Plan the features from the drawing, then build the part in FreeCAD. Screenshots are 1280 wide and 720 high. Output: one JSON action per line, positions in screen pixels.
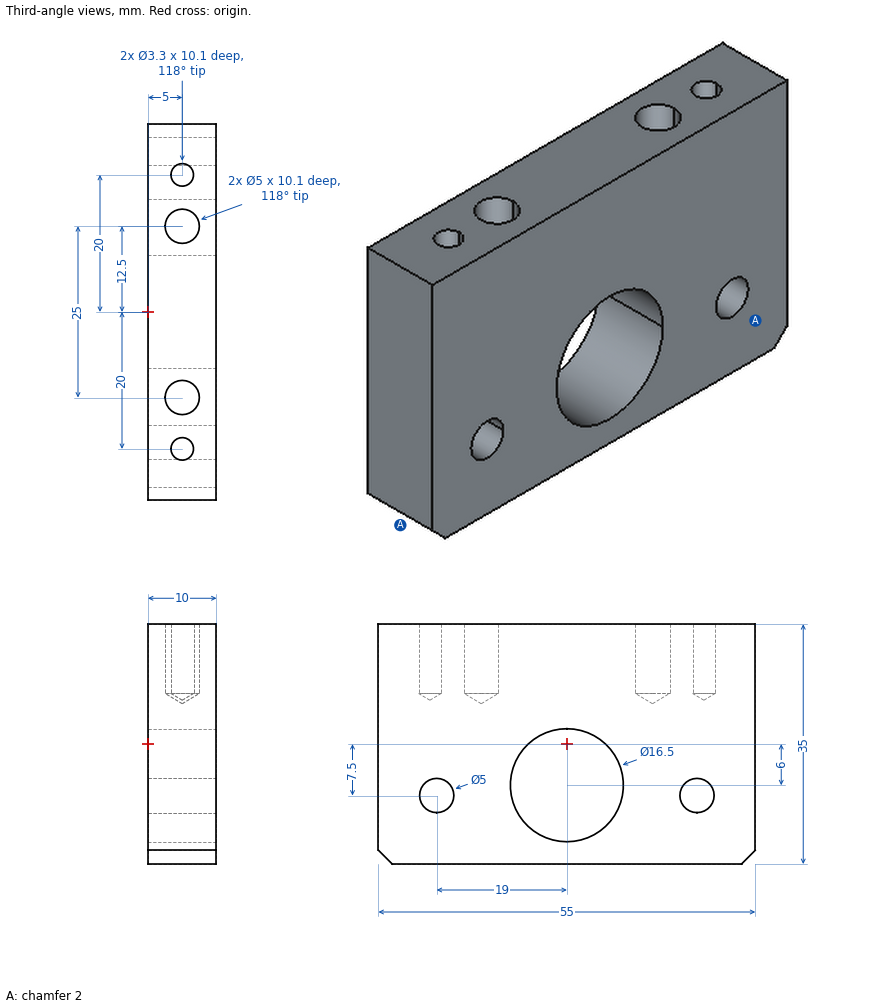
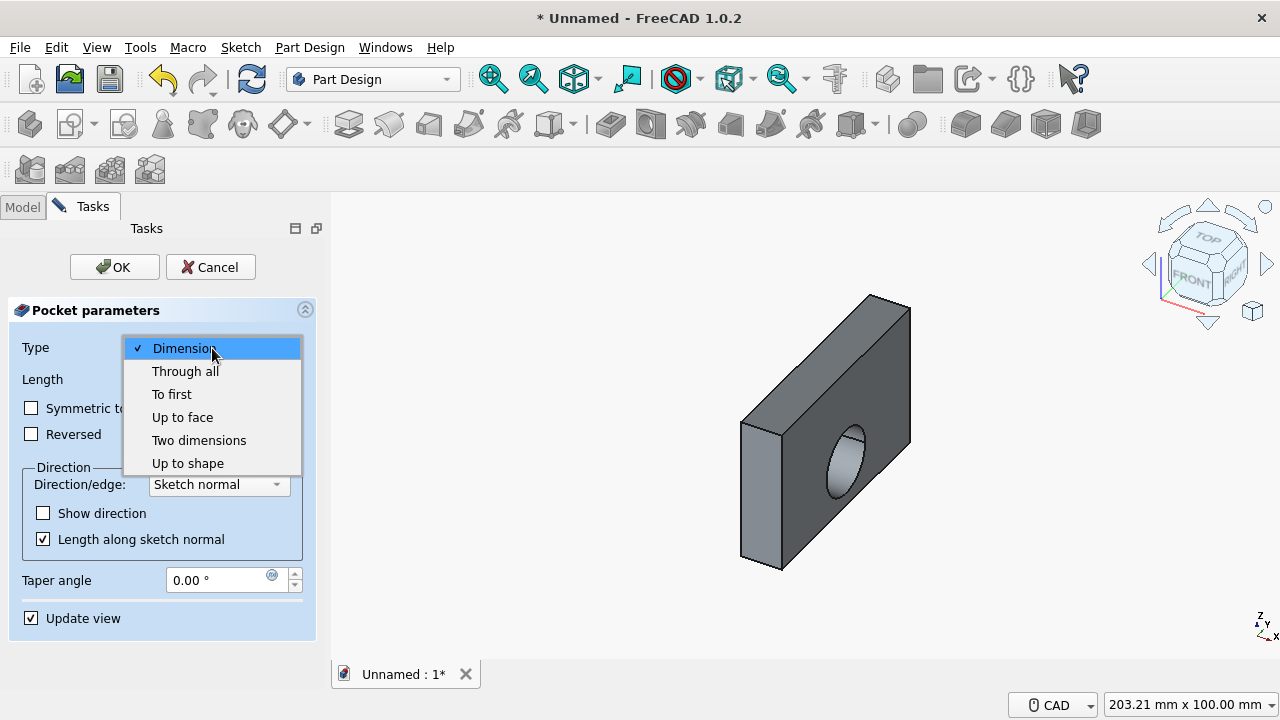
{"action": "left_click", "coordinate": [212, 372]}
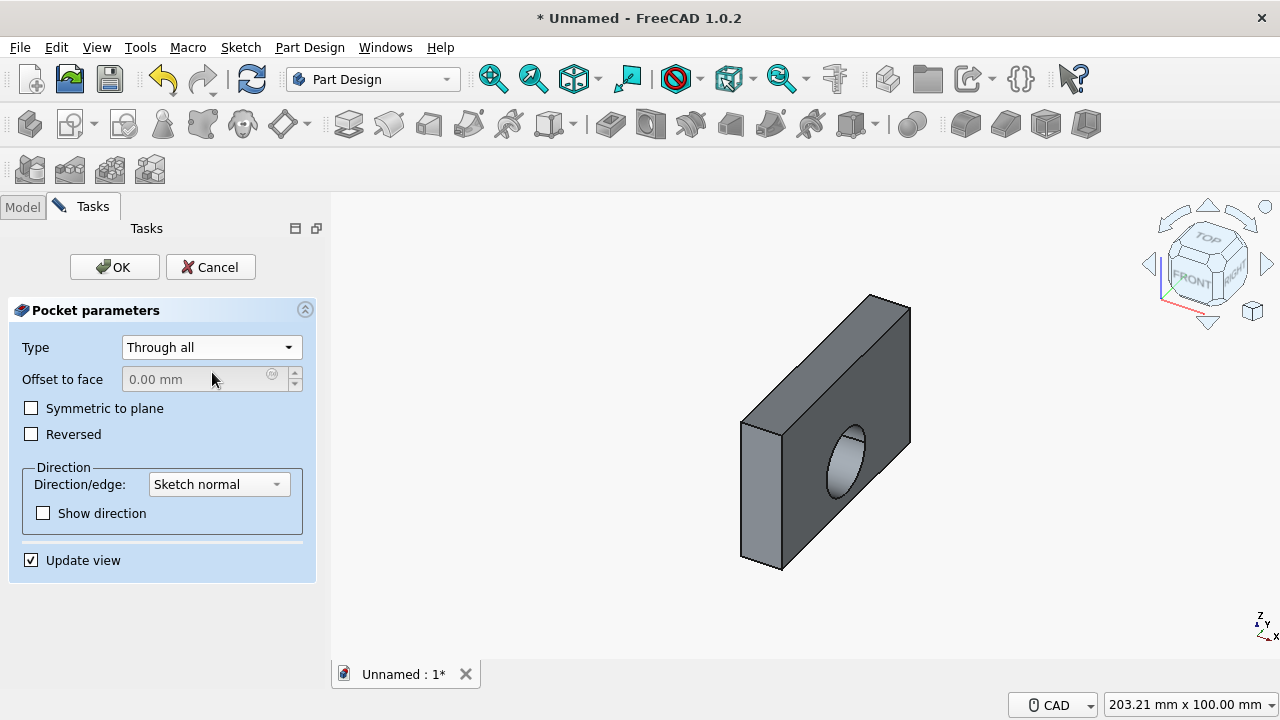
{"action": "left_click", "coordinate": [30, 434]}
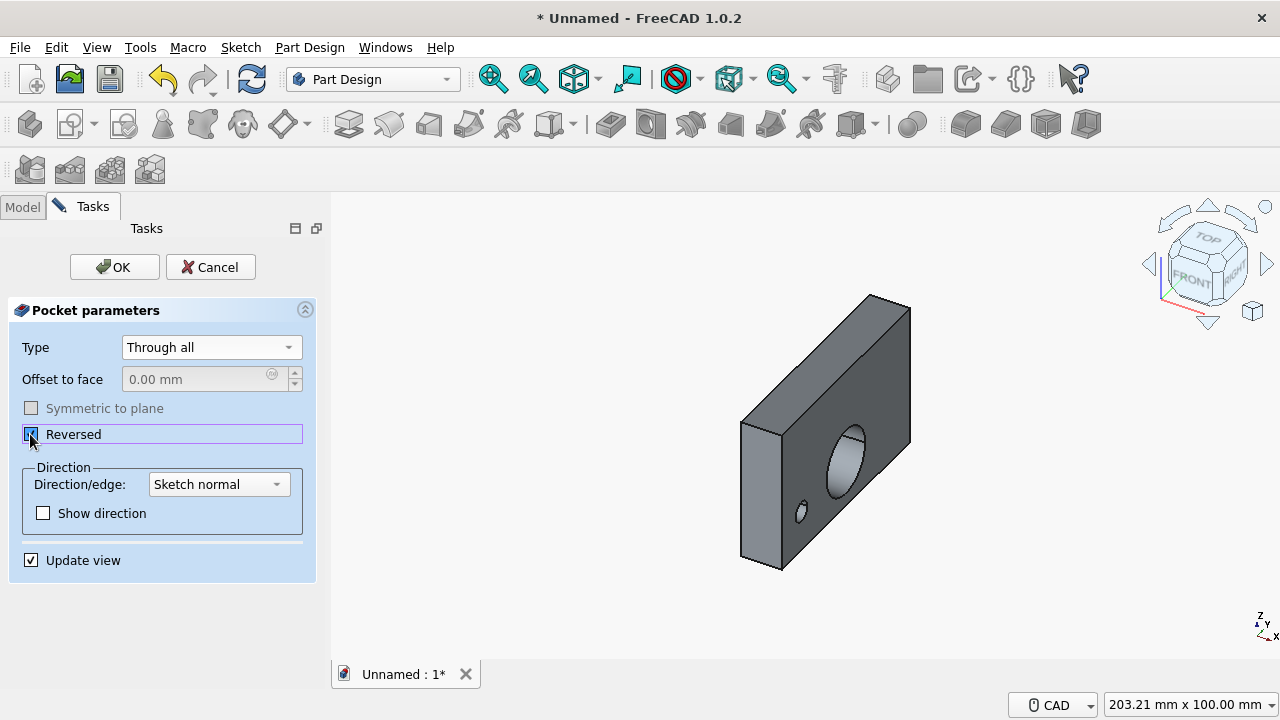
{"action": "left_click", "coordinate": [115, 267]}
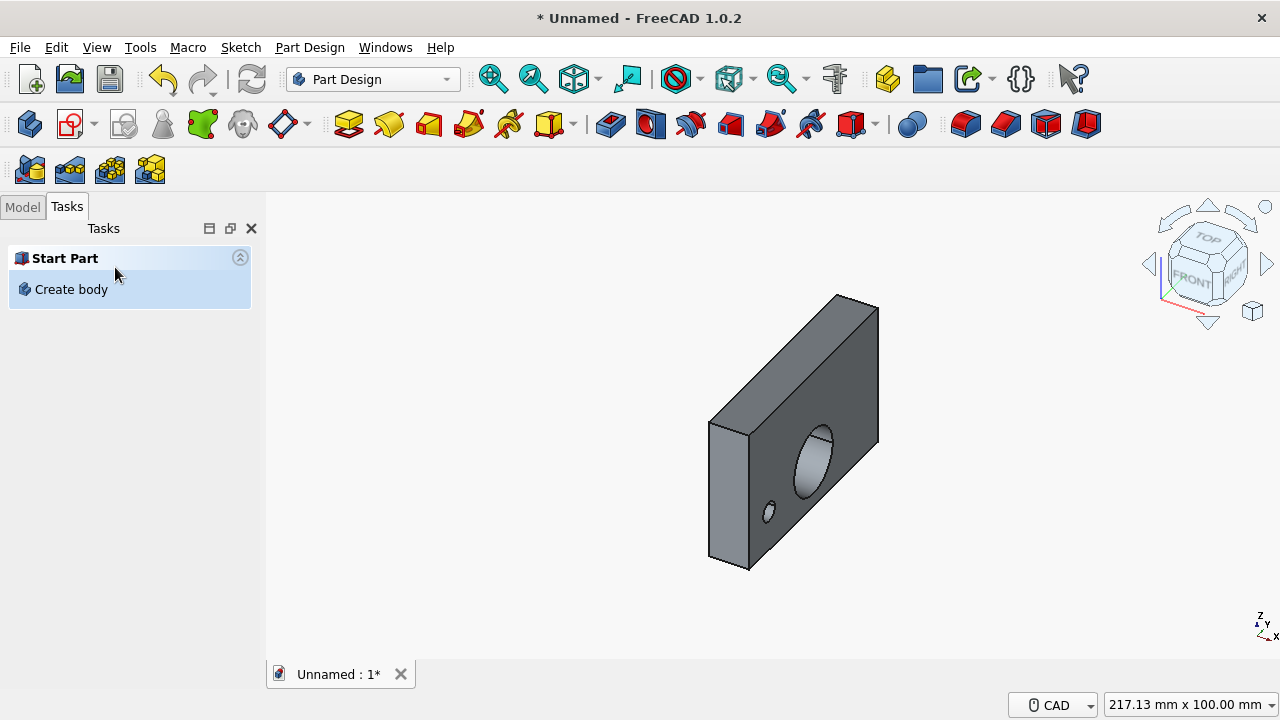
{"action": "left_click", "coordinate": [23, 206]}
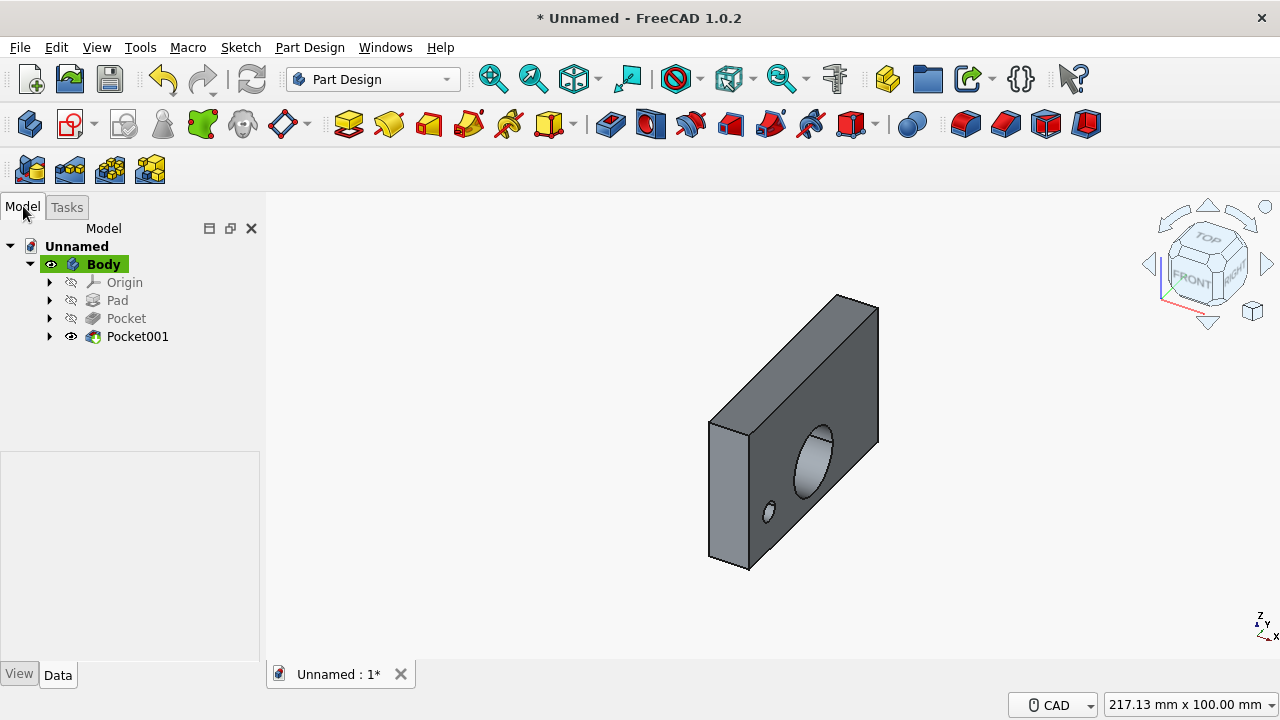
{"action": "left_click", "coordinate": [116, 336]}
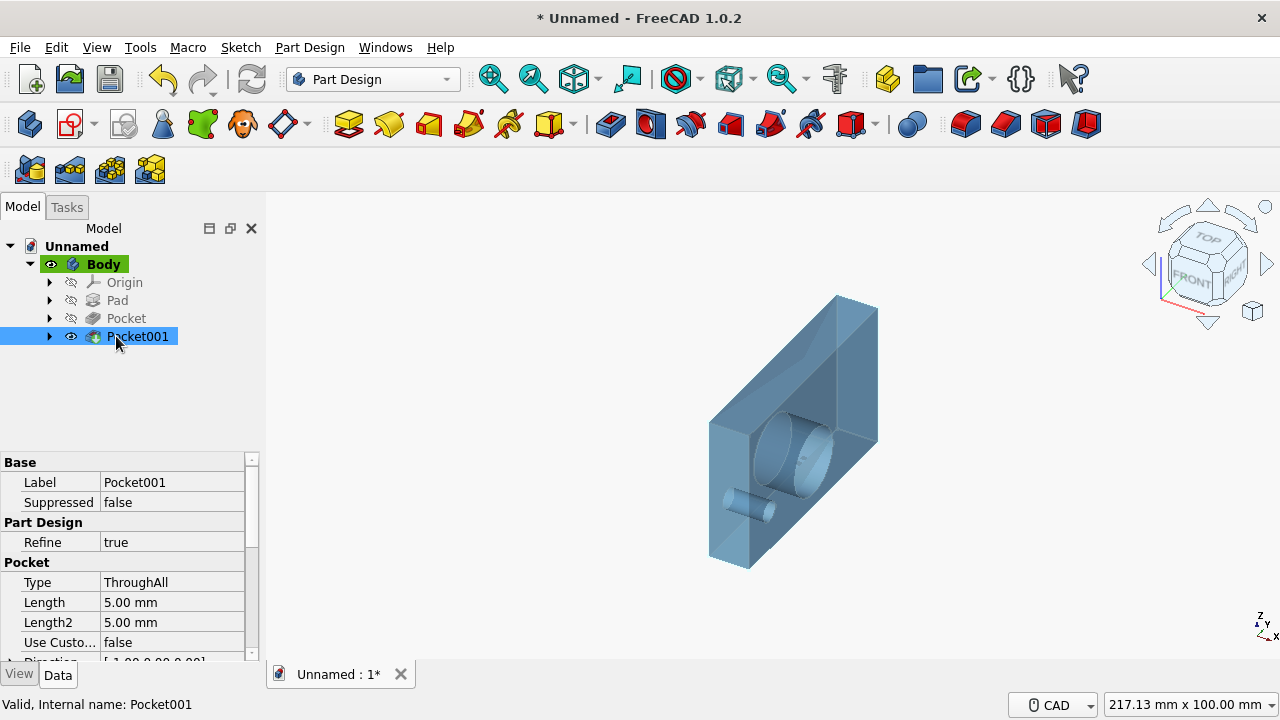
{"action": "left_click", "coordinate": [30, 170]}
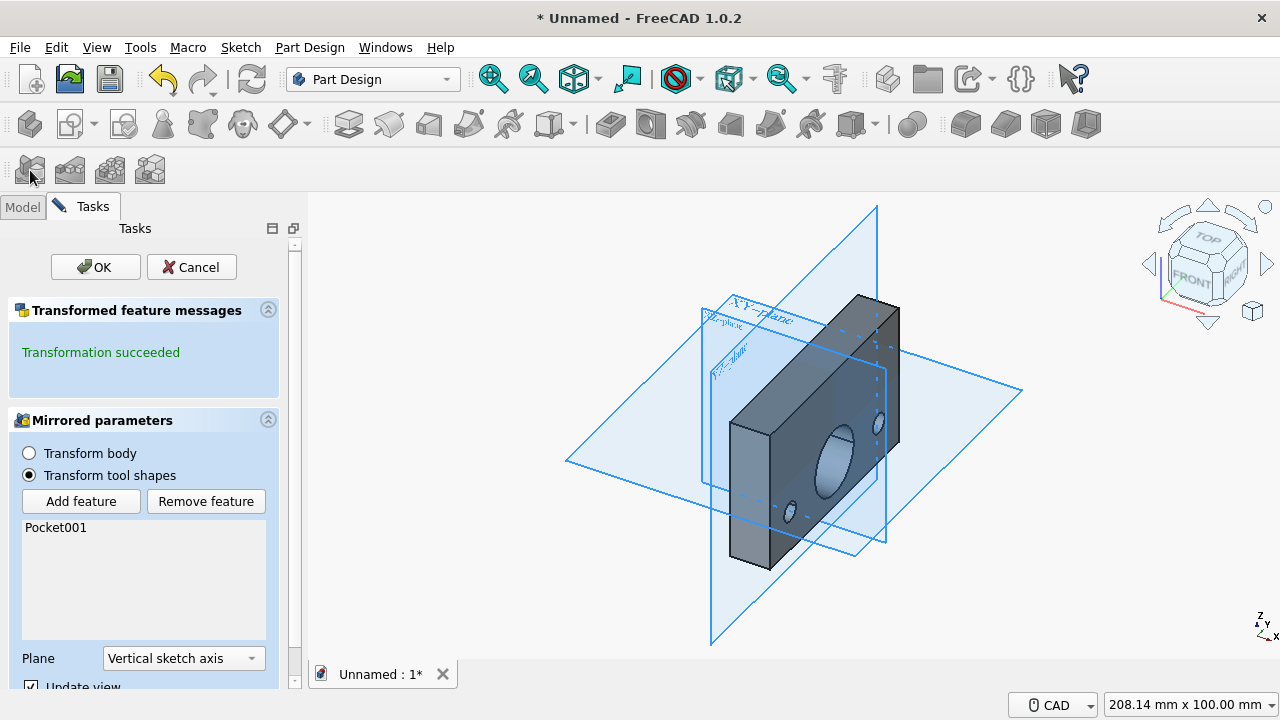
{"action": "left_click", "coordinate": [184, 658]}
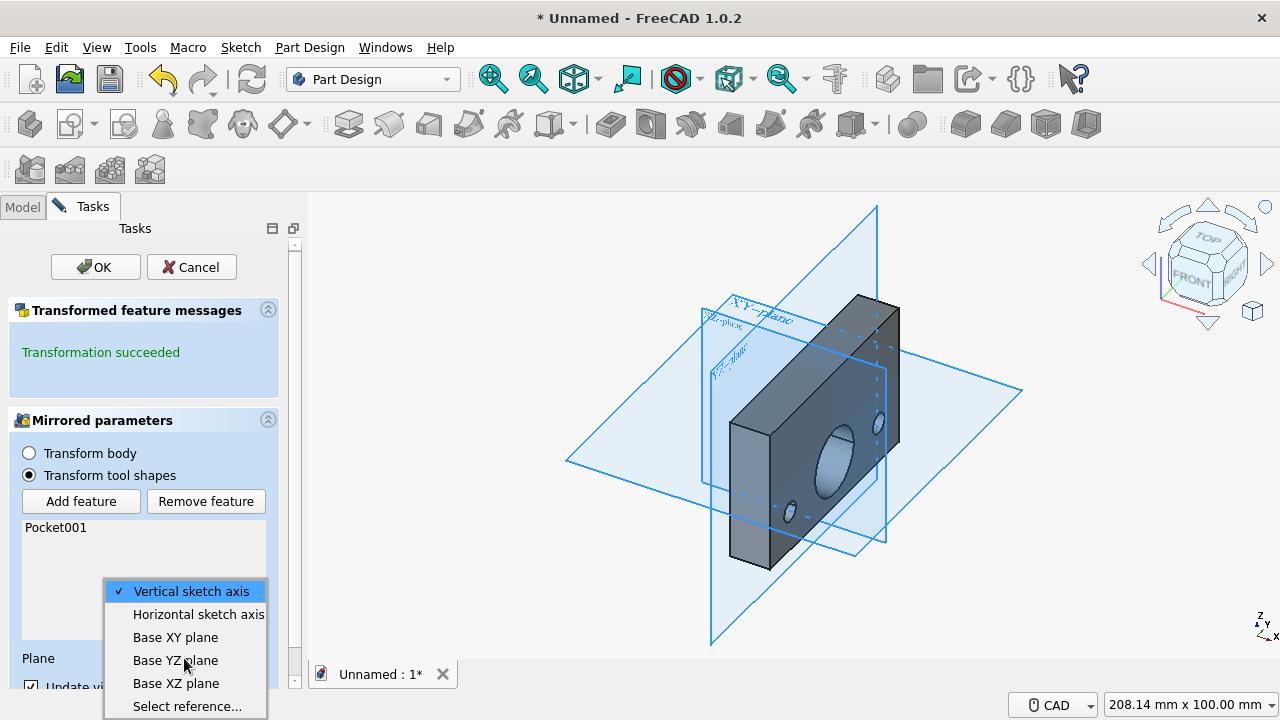
{"action": "left_click", "coordinate": [184, 684]}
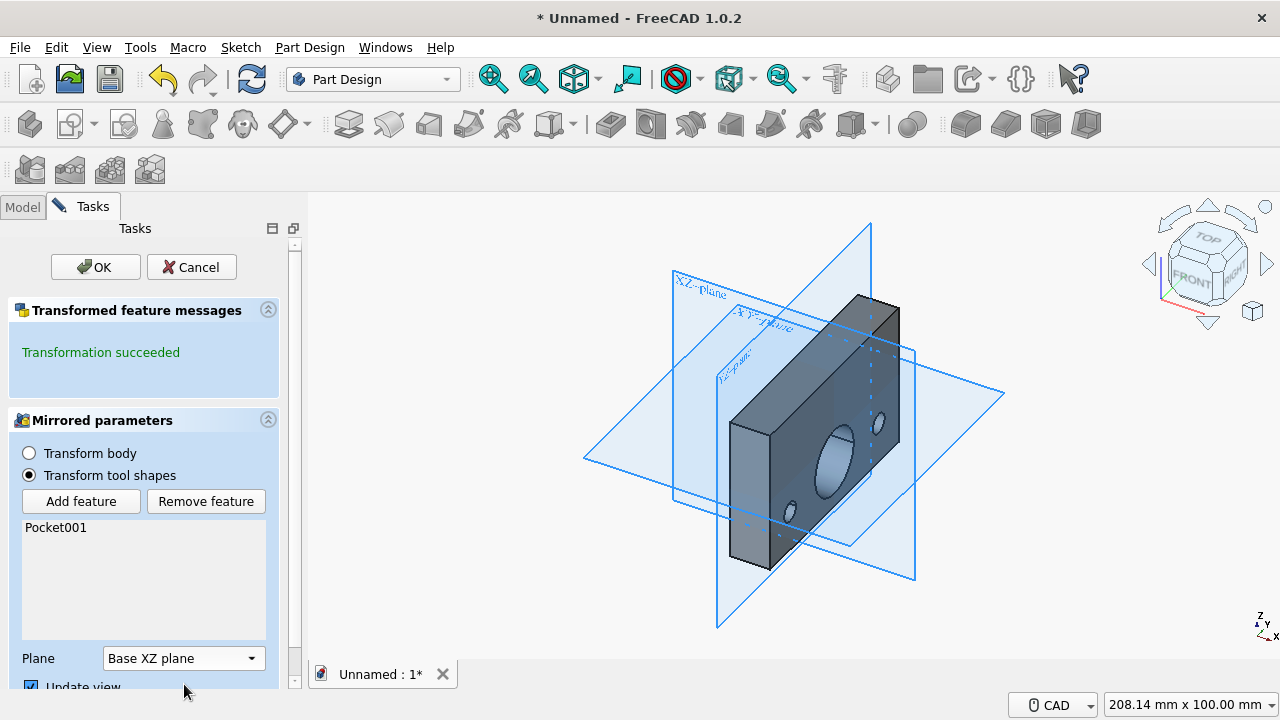
{"action": "left_click", "coordinate": [96, 267]}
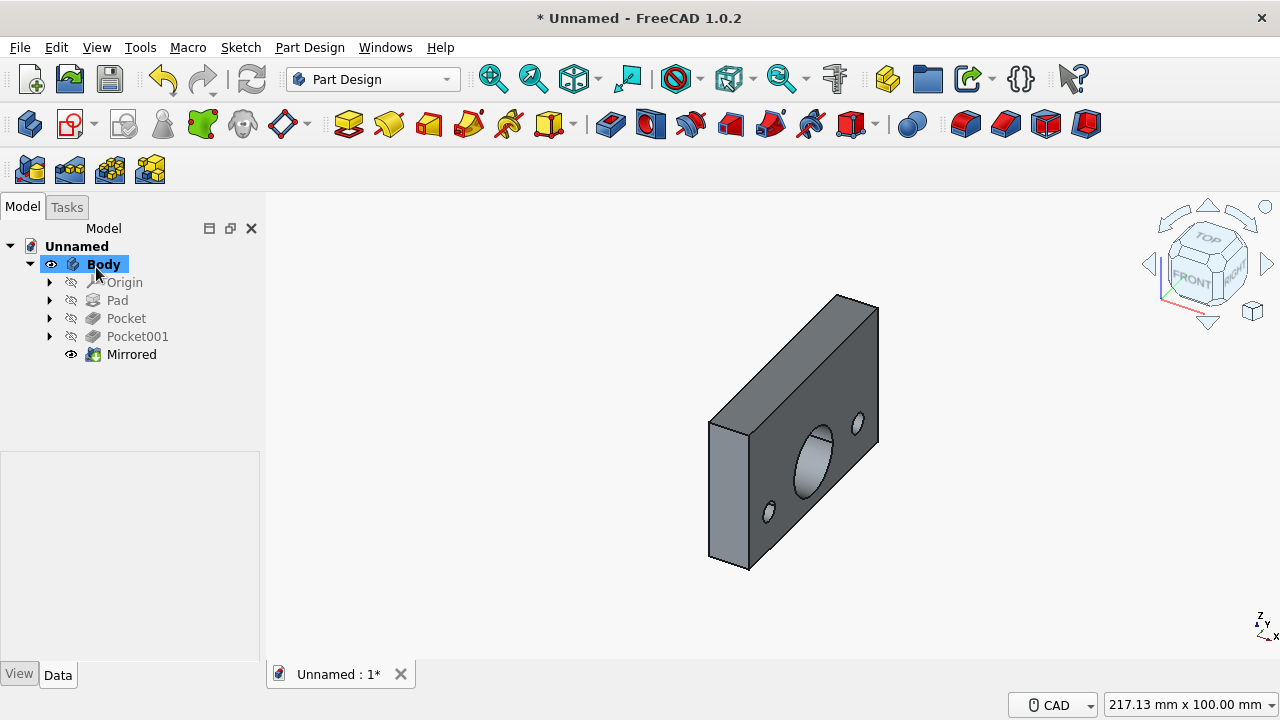
{"action": "left_click", "coordinate": [830, 328]}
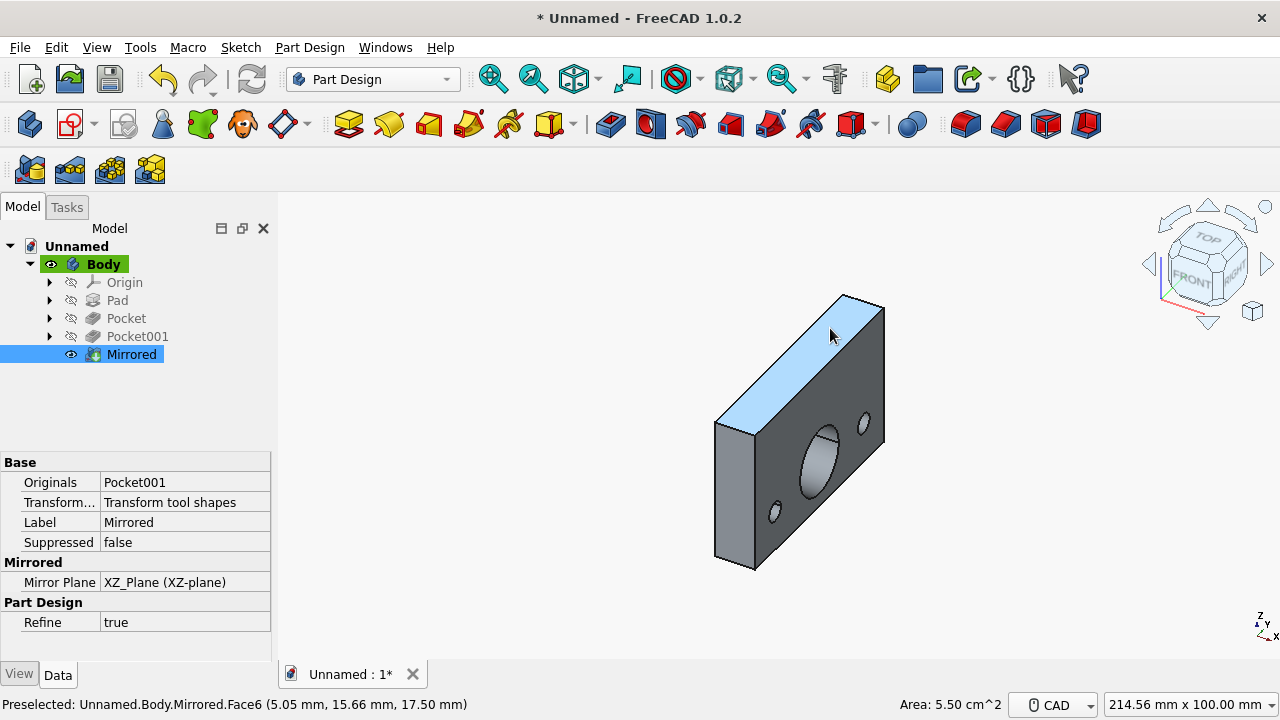
{"action": "left_click", "coordinate": [70, 124]}